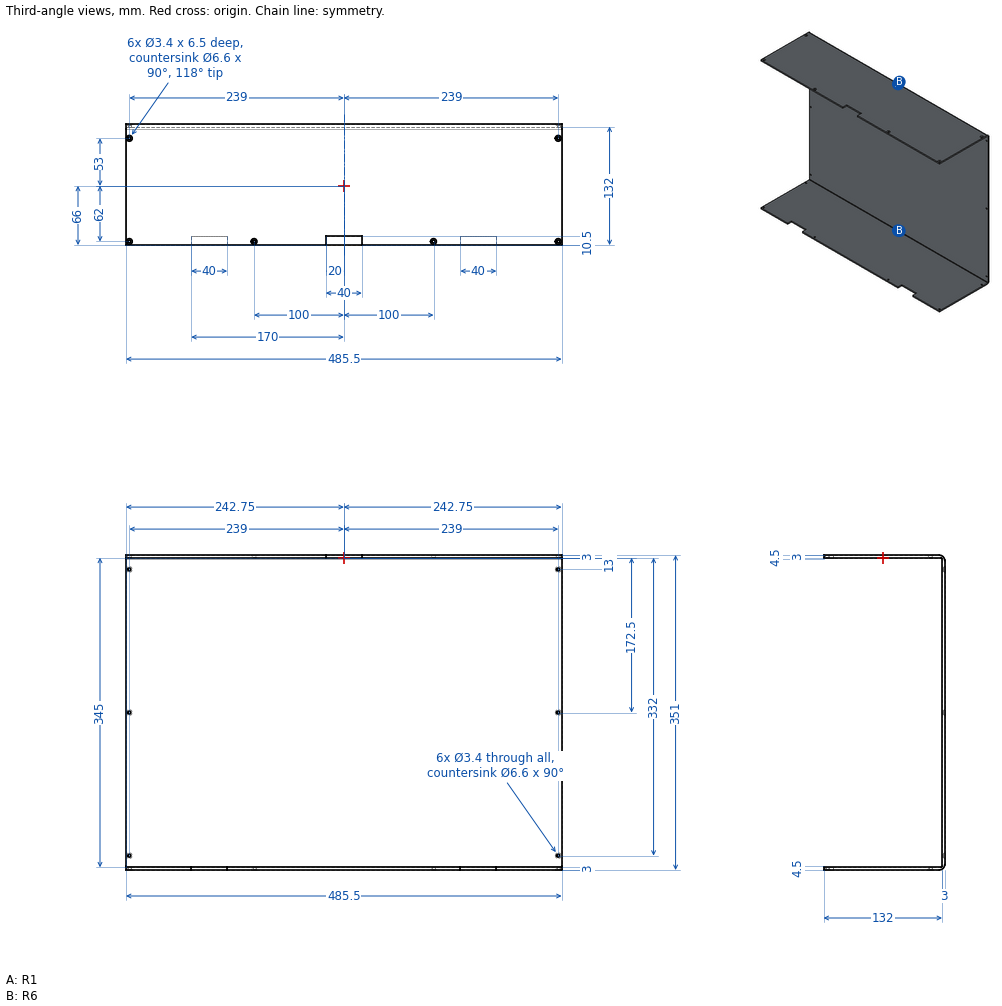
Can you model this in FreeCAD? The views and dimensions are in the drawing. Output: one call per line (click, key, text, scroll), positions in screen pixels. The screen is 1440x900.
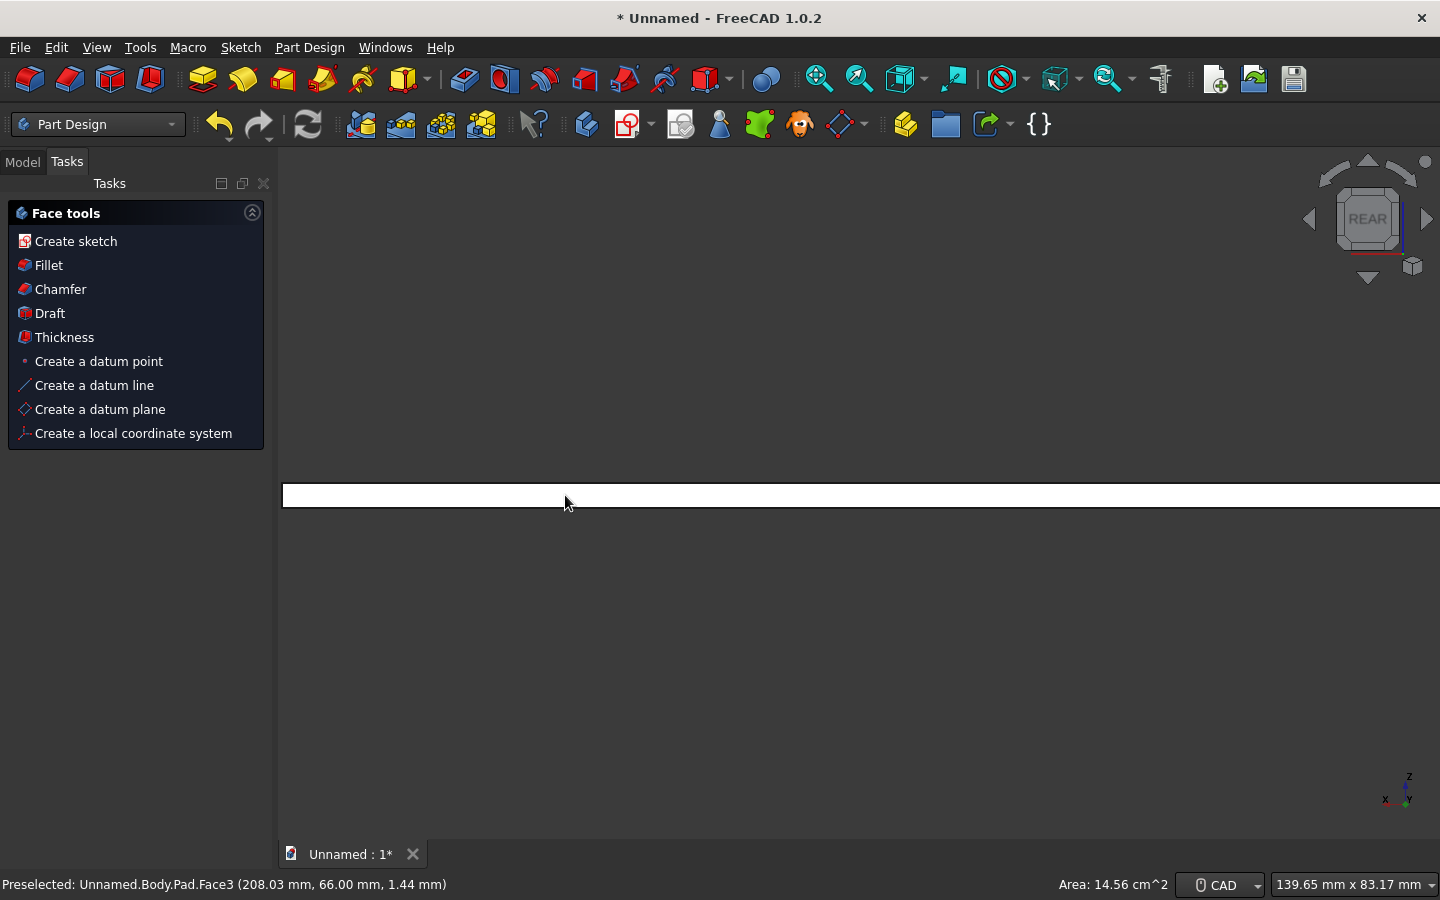
click(628, 124)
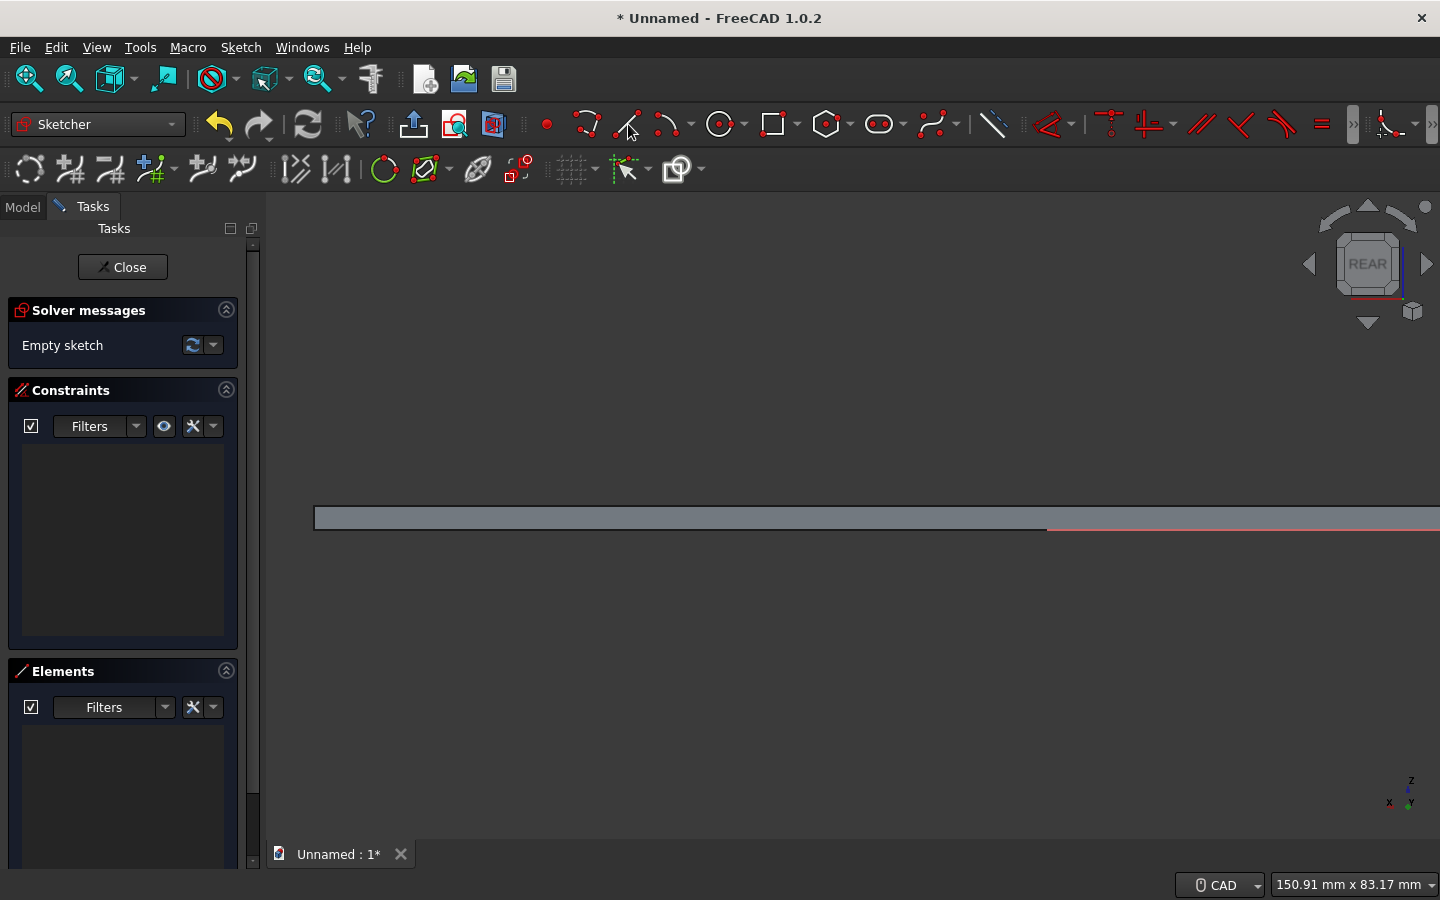
scroll(504, 247, down, 9)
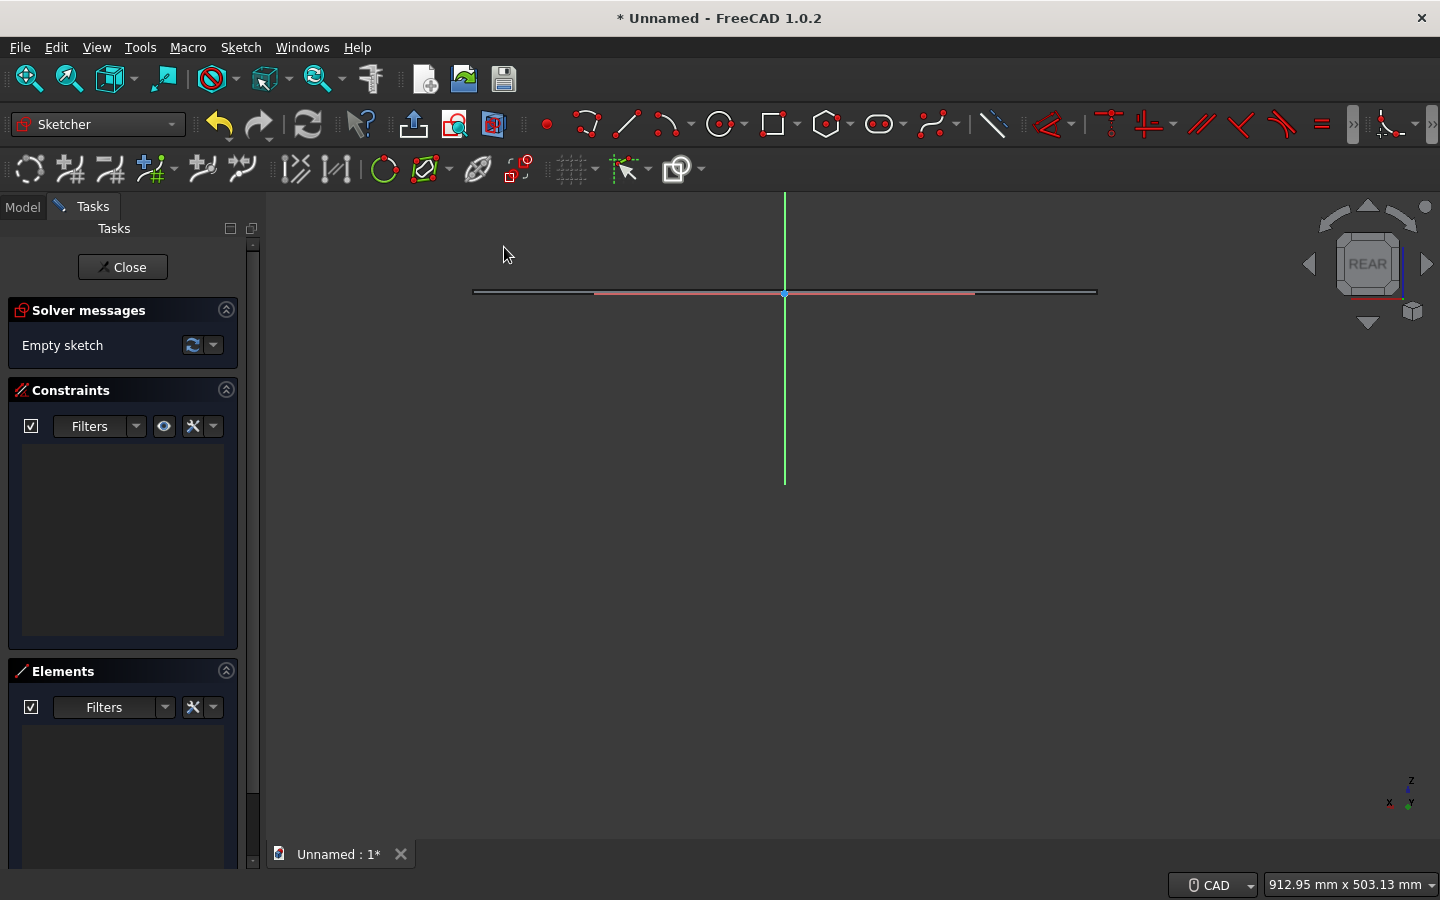
click(774, 124)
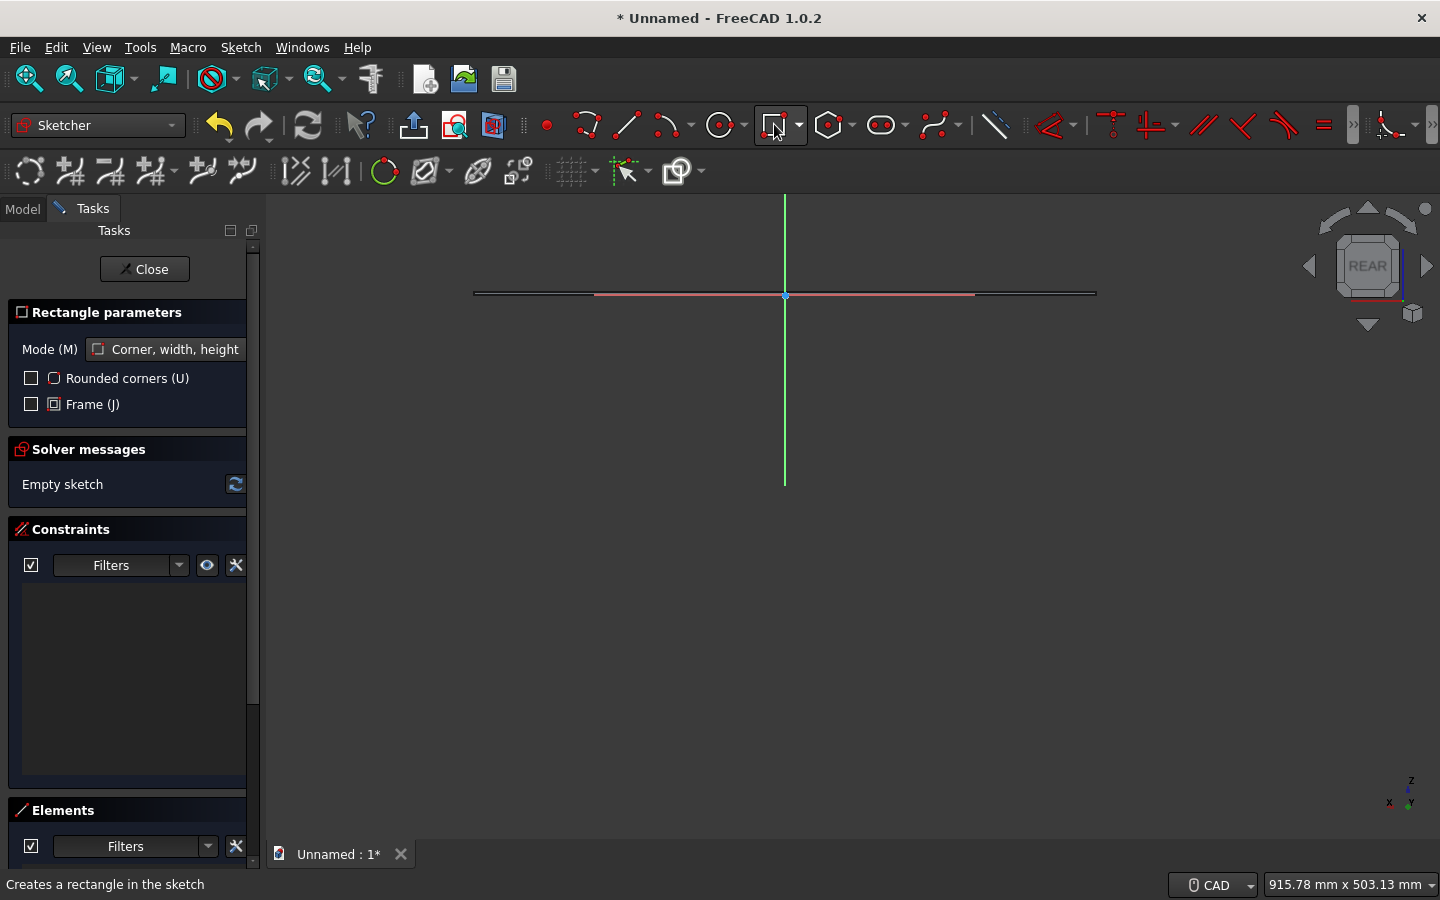
scroll(474, 292, up, 8)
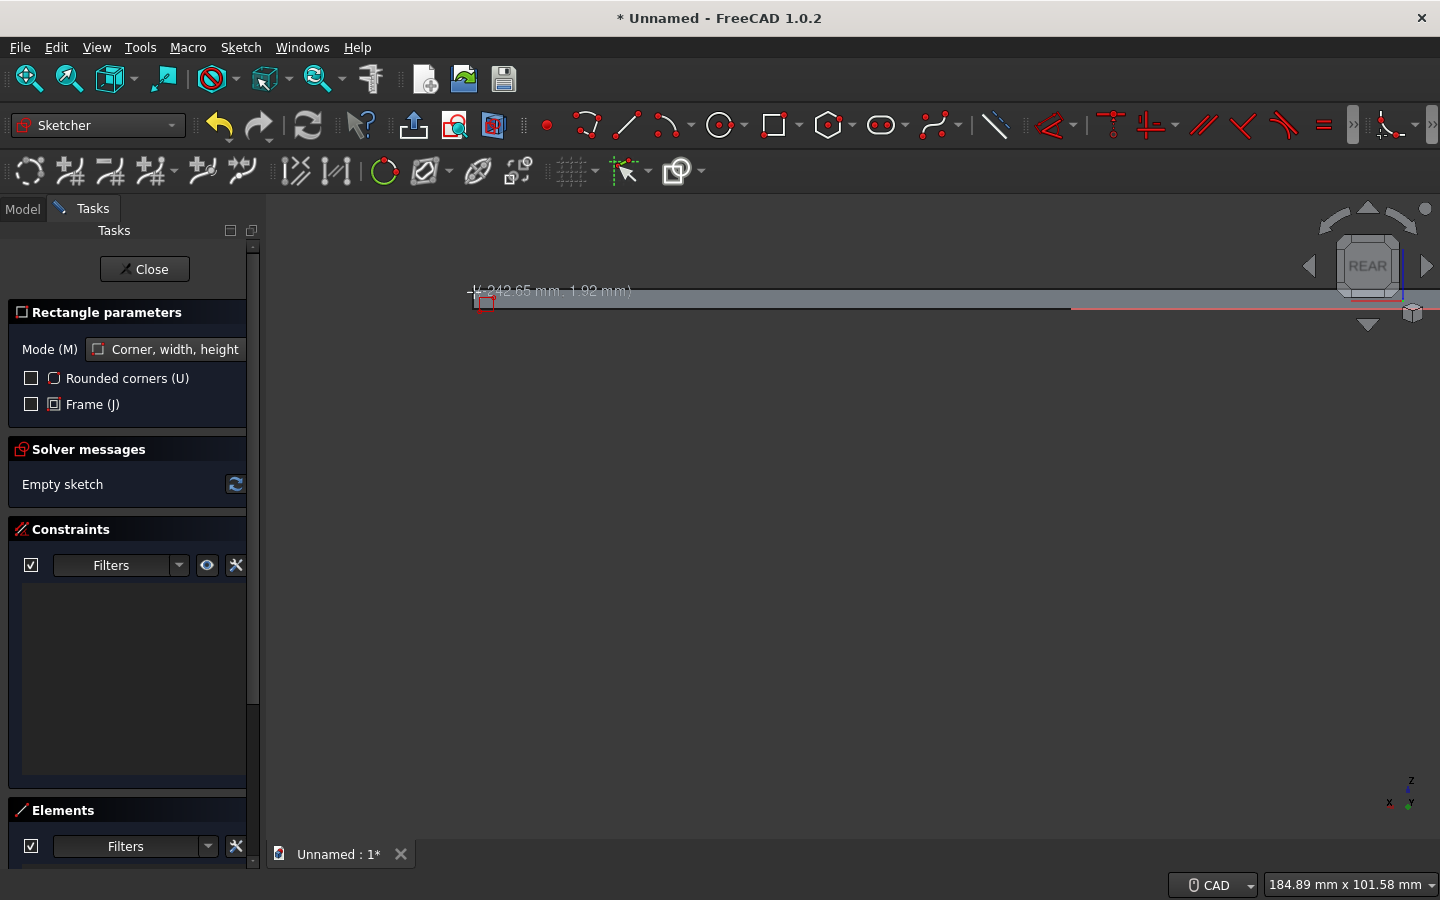
click(473, 289)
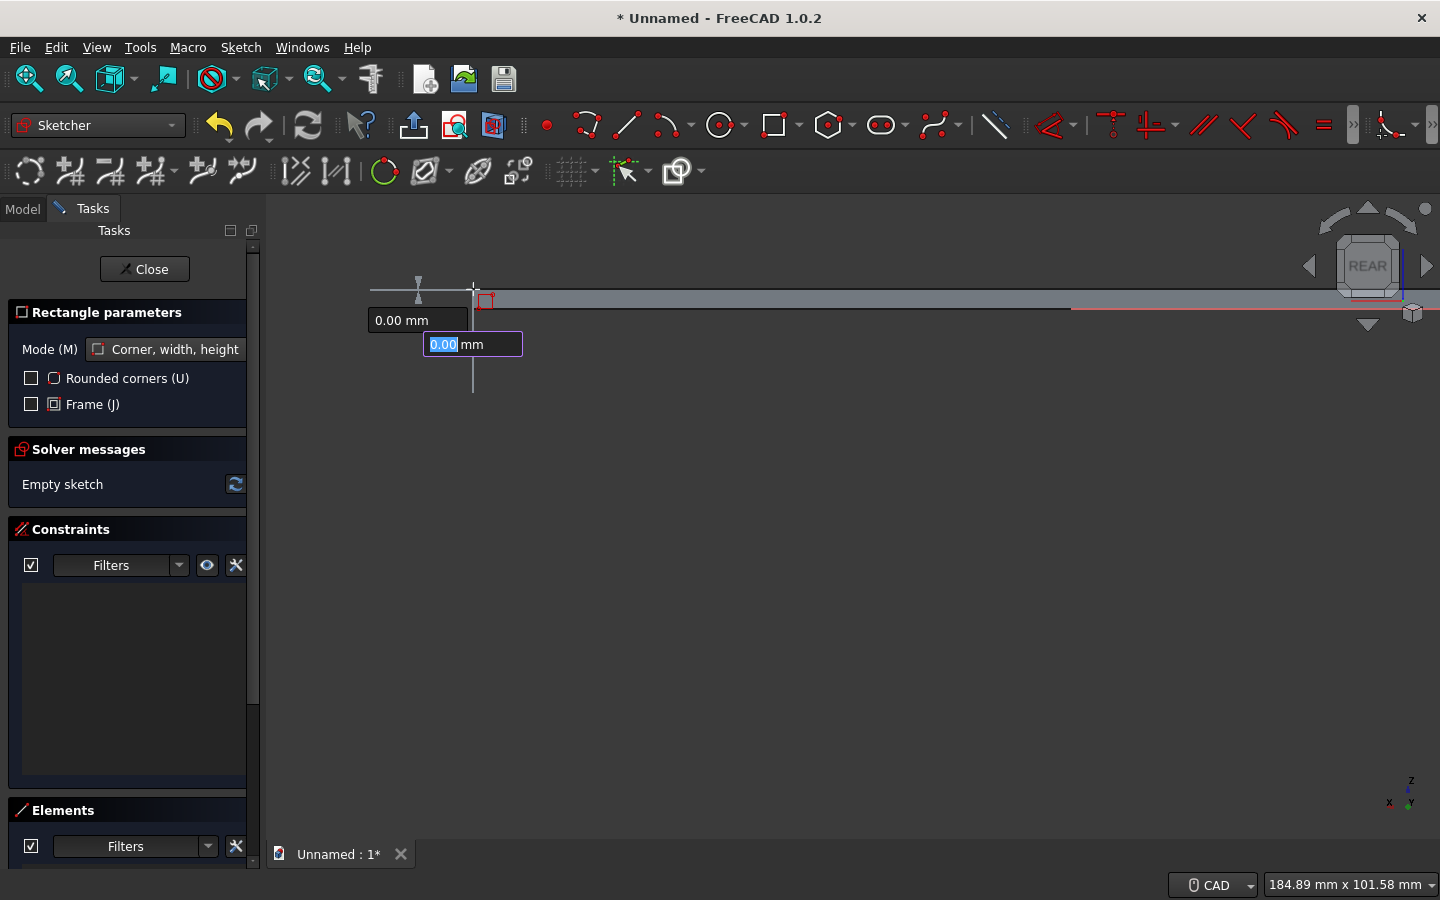
scroll(473, 292, down, 8)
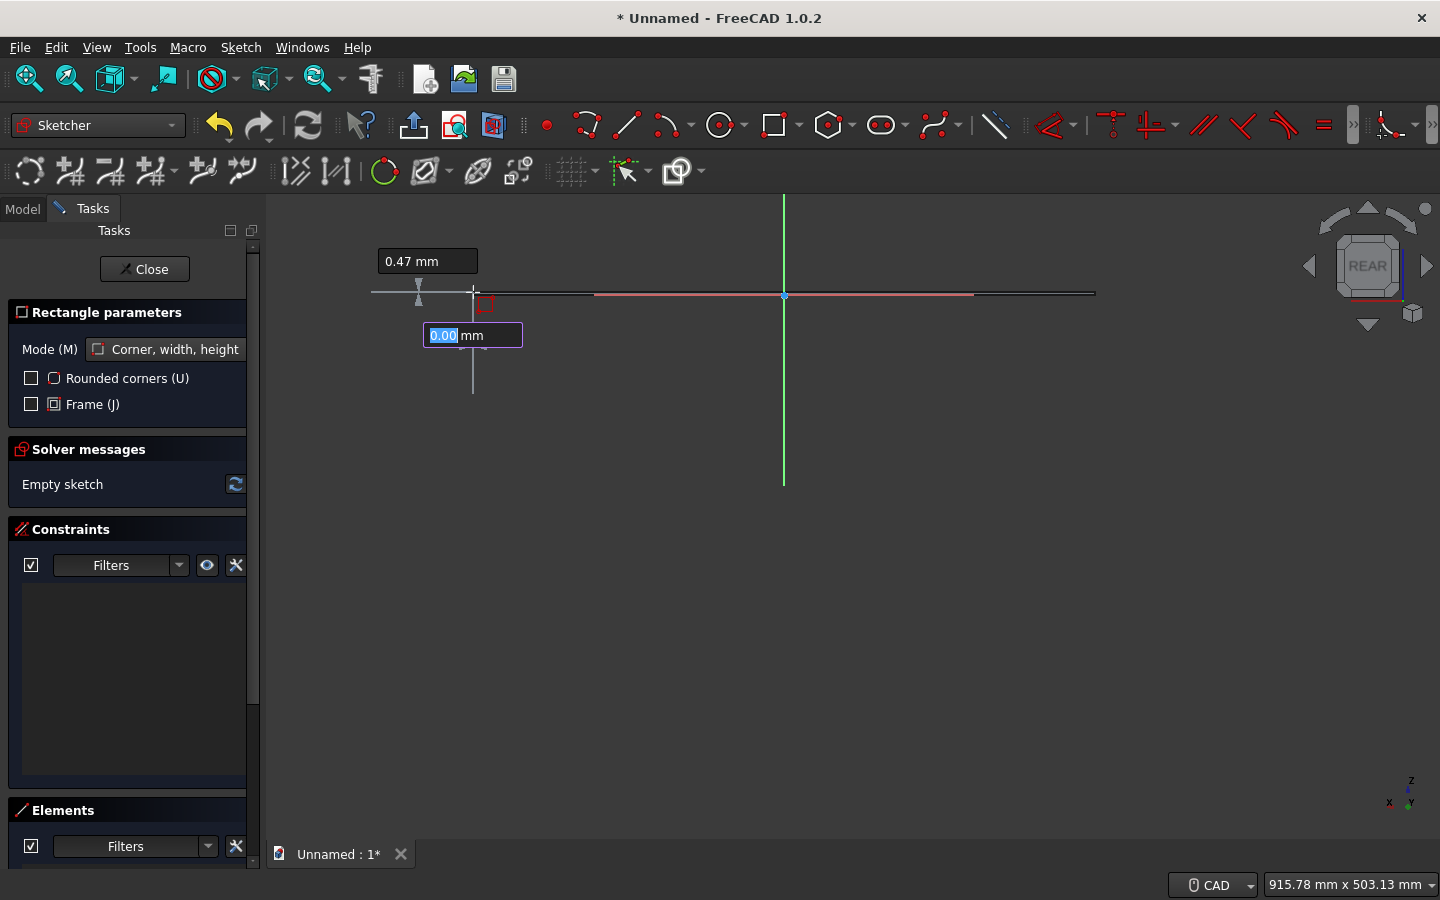
click(1095, 742)
key(Escape)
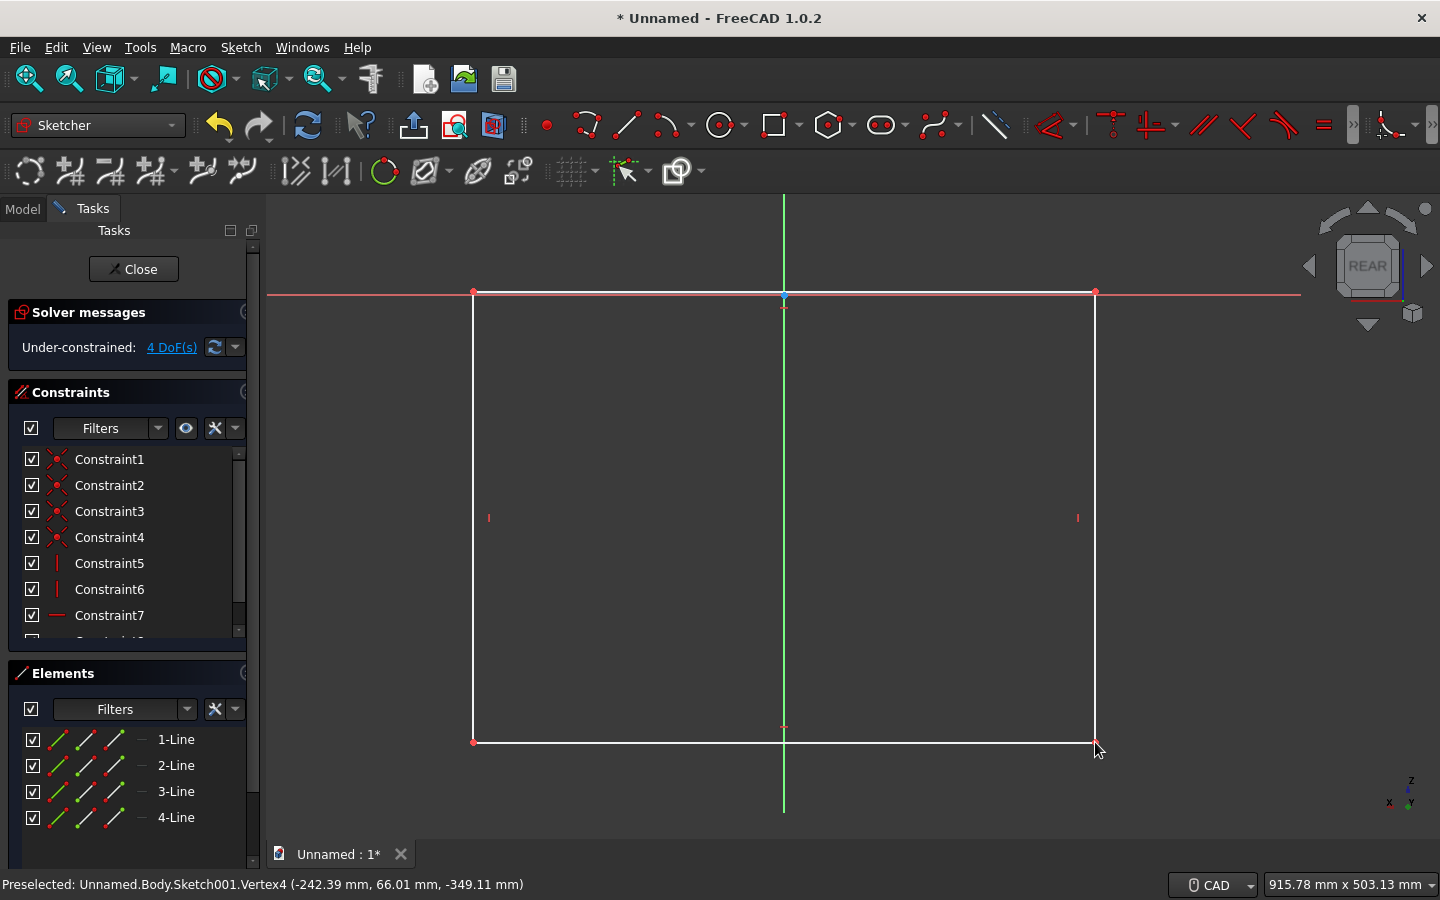
scroll(473, 292, up, 12)